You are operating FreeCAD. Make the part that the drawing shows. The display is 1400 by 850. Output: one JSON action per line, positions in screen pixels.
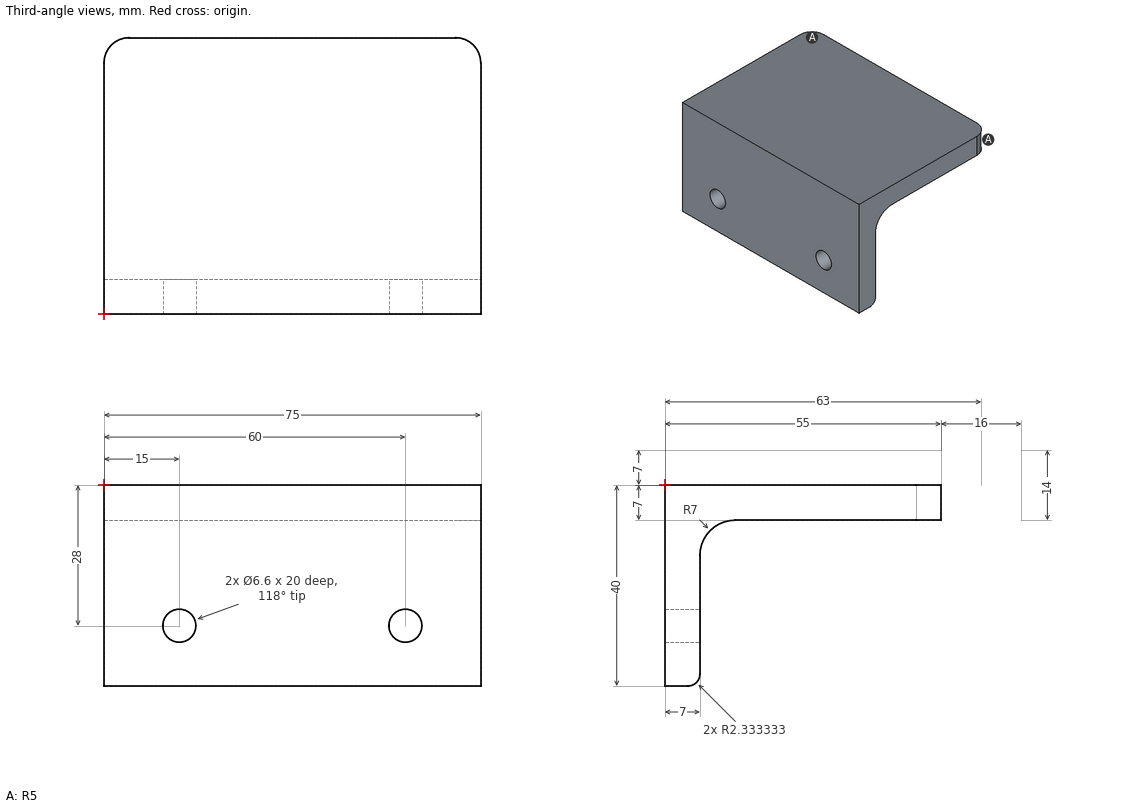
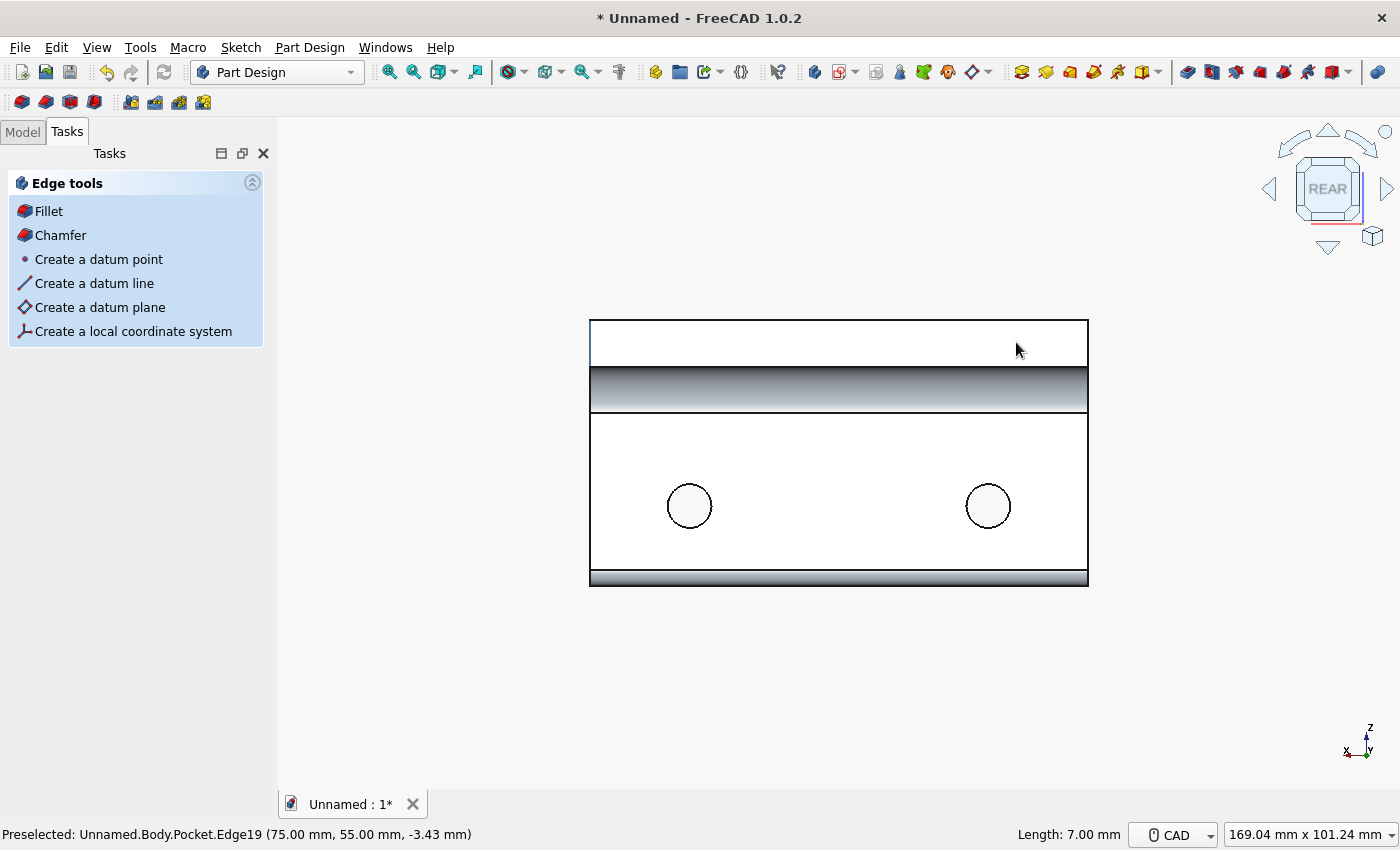
{"action": "left_click", "coordinate": [390, 72]}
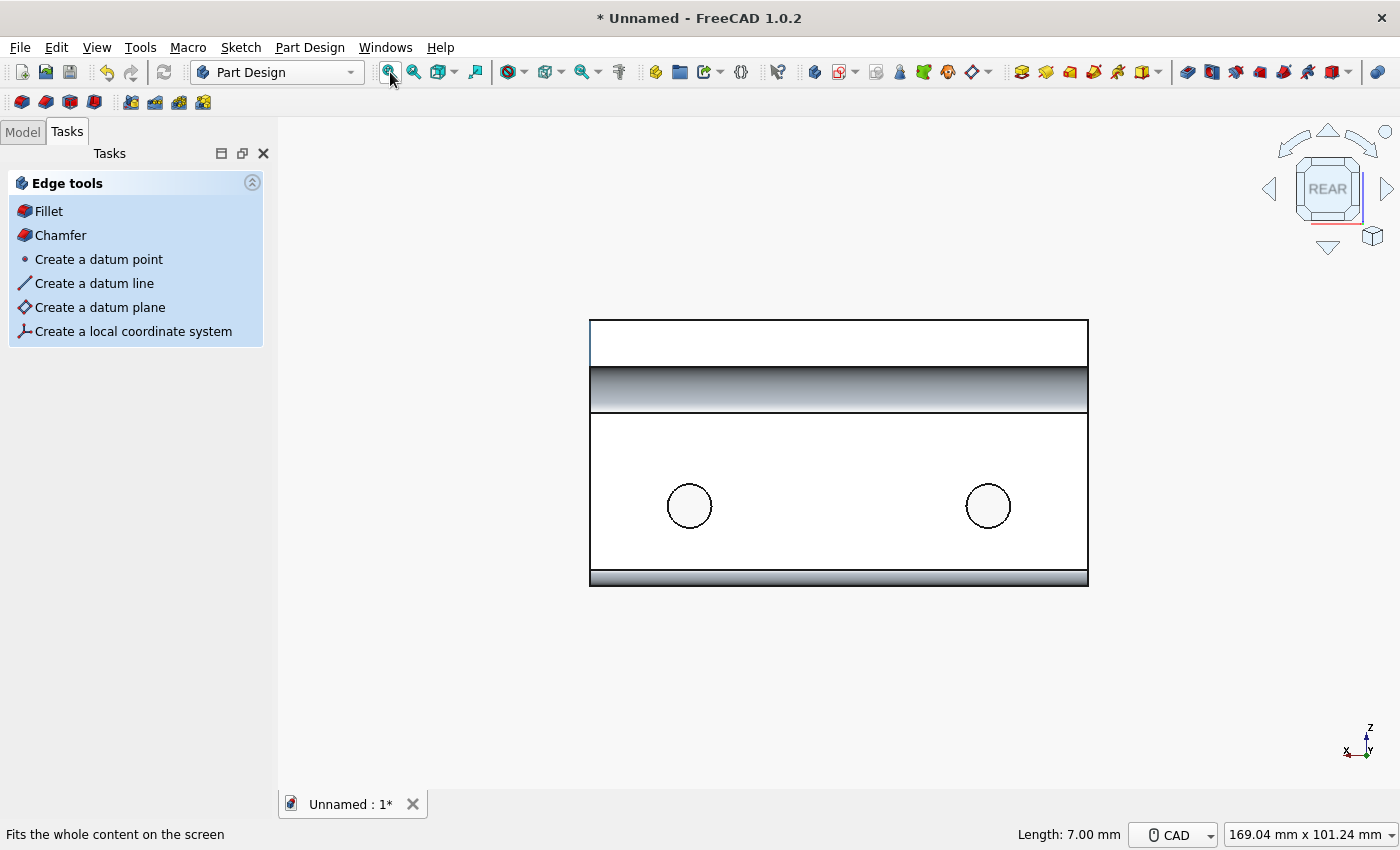
{"action": "left_click", "coordinate": [1088, 342], "text": "ctrl"}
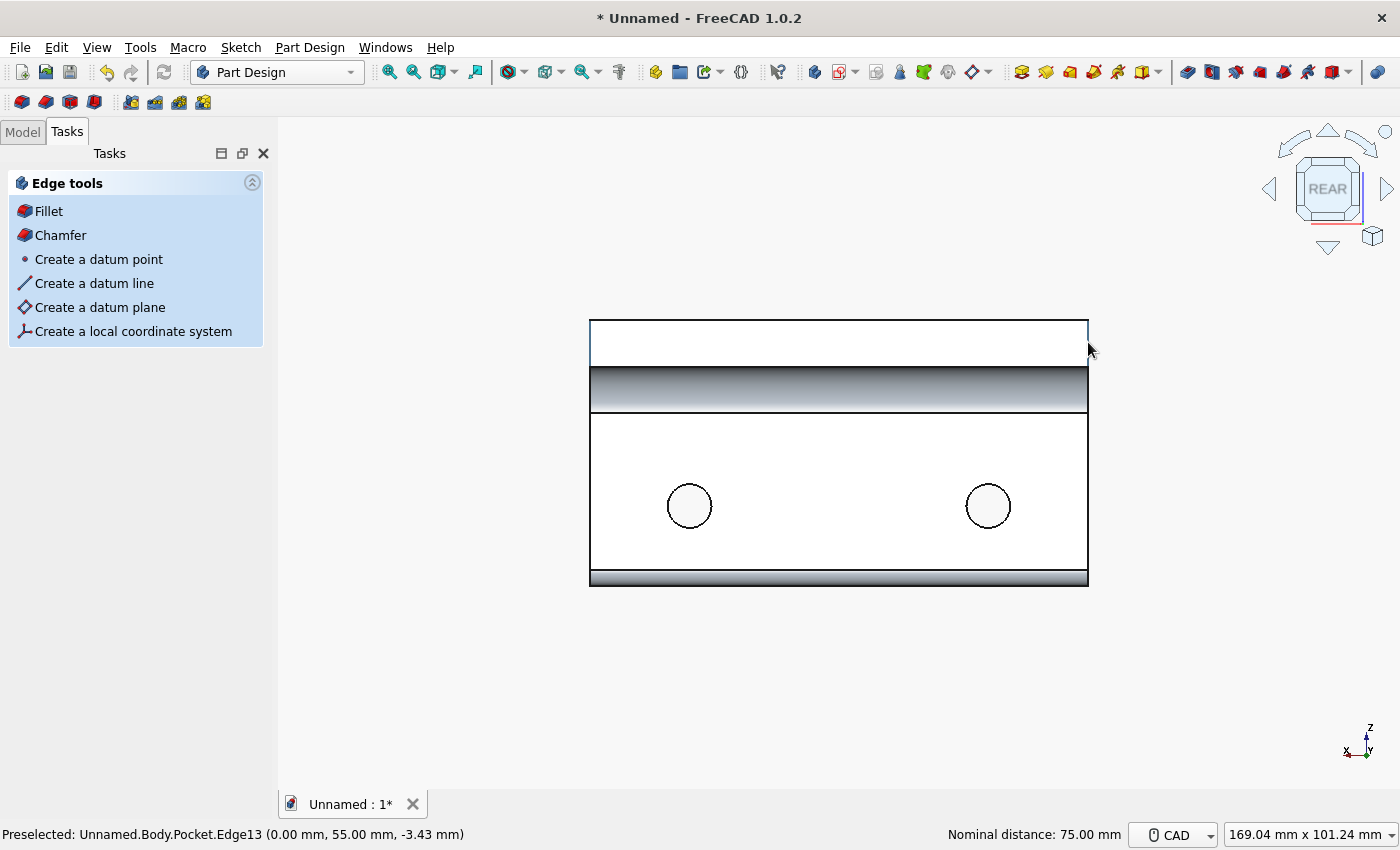
{"action": "left_click", "coordinate": [22, 102]}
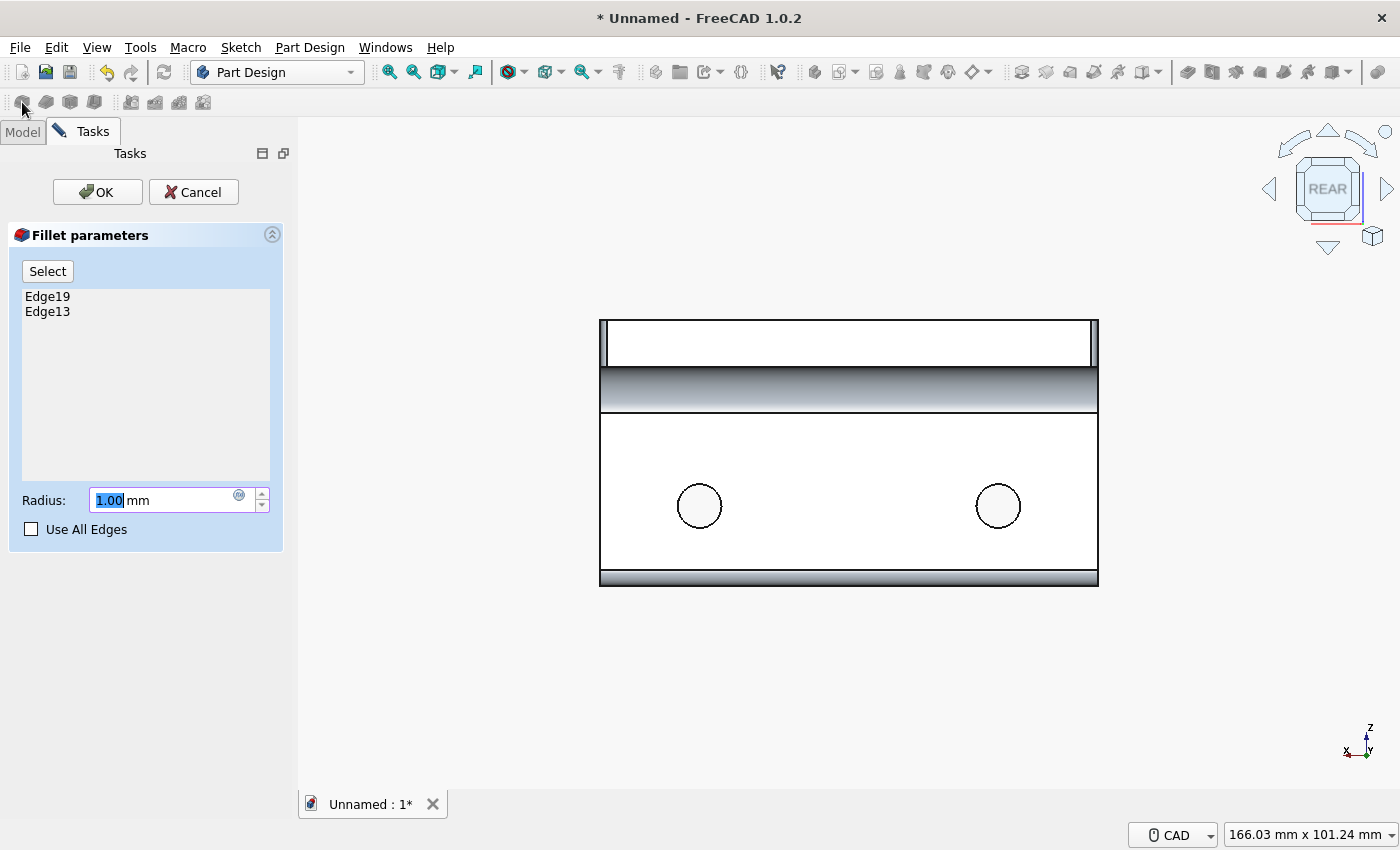
{"action": "type", "text": "5"}
{"action": "key", "text": "Tab"}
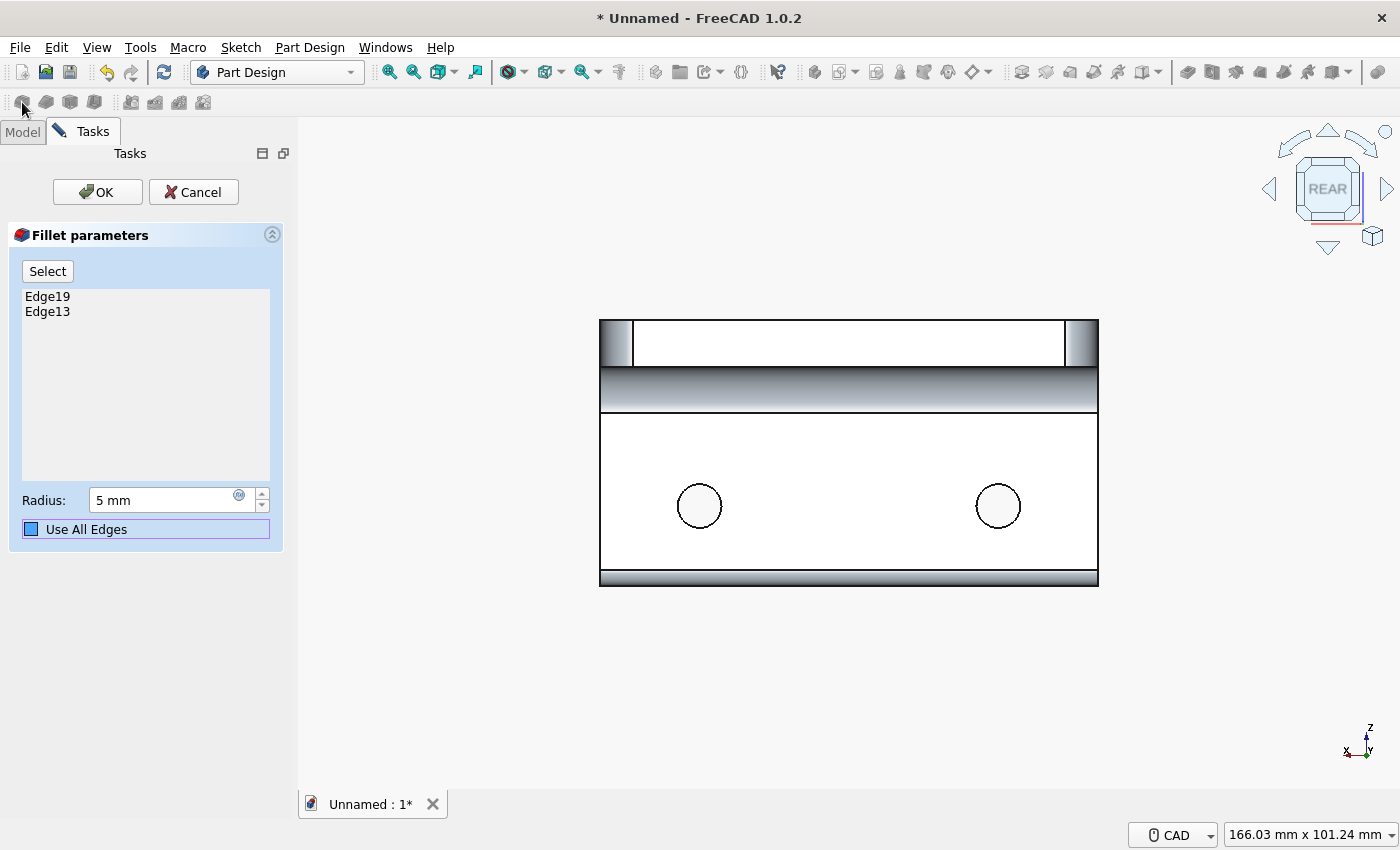
{"action": "left_click", "coordinate": [98, 192]}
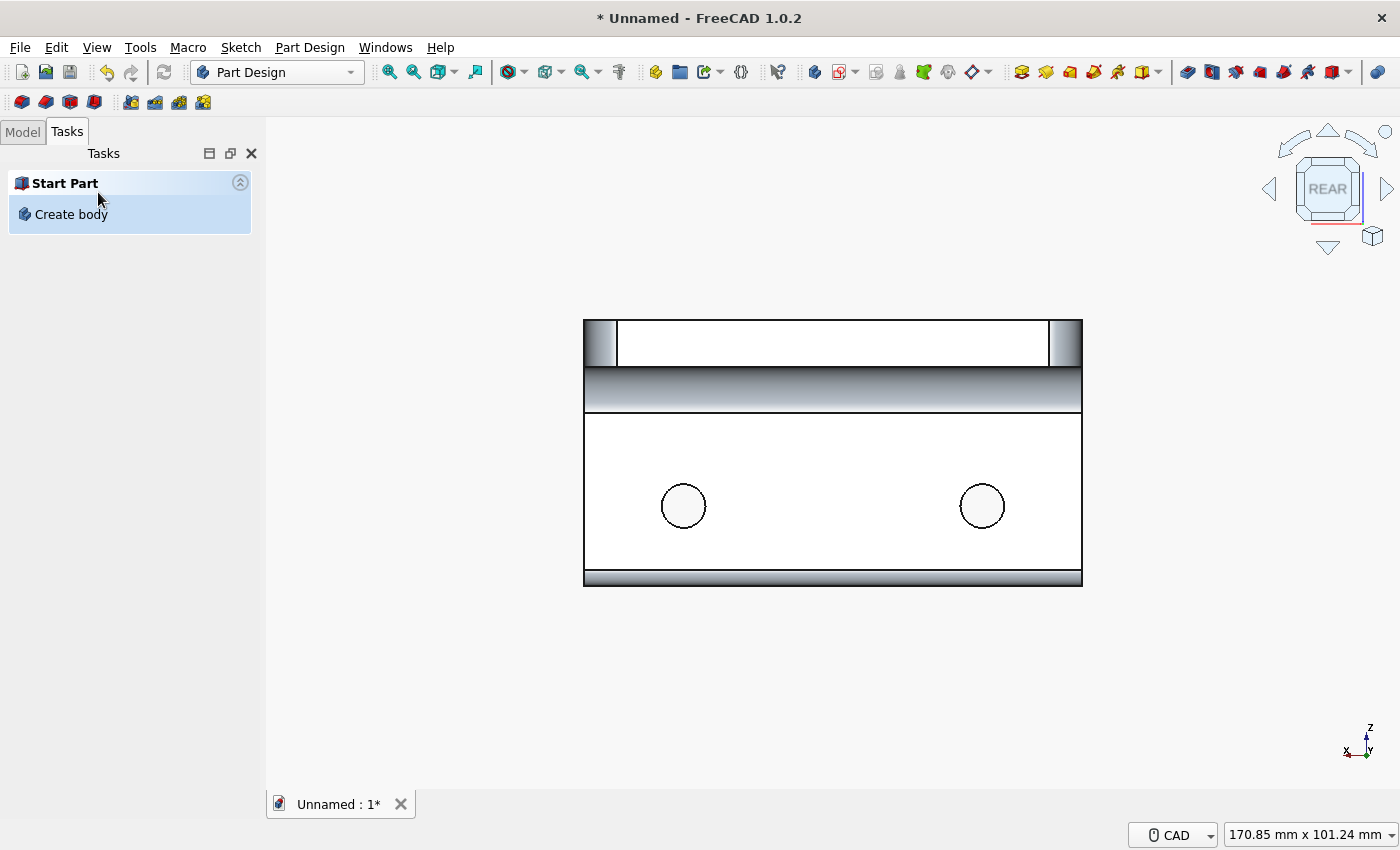
{"action": "key", "text": "0"}